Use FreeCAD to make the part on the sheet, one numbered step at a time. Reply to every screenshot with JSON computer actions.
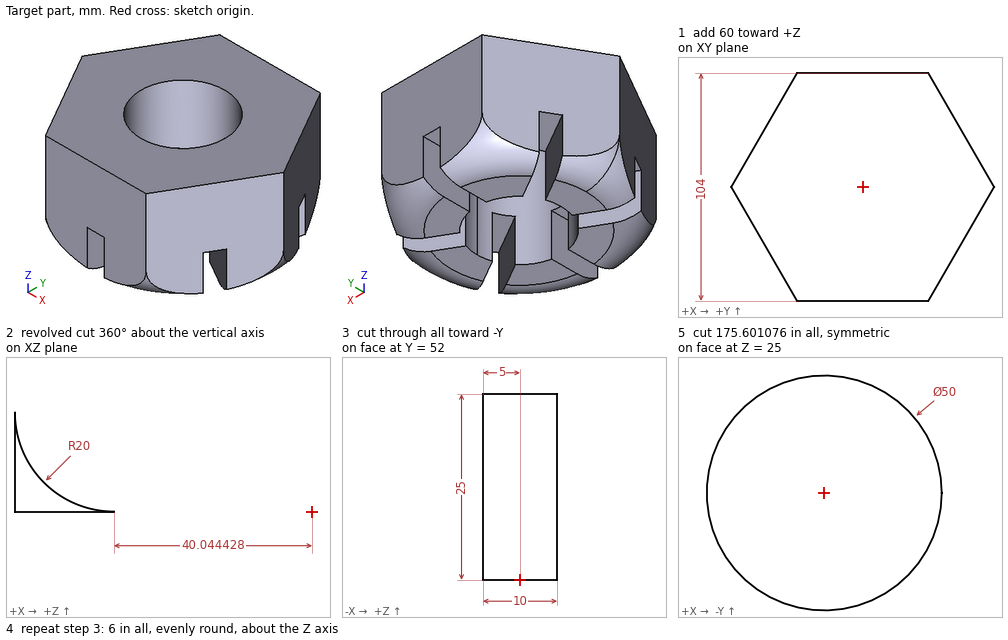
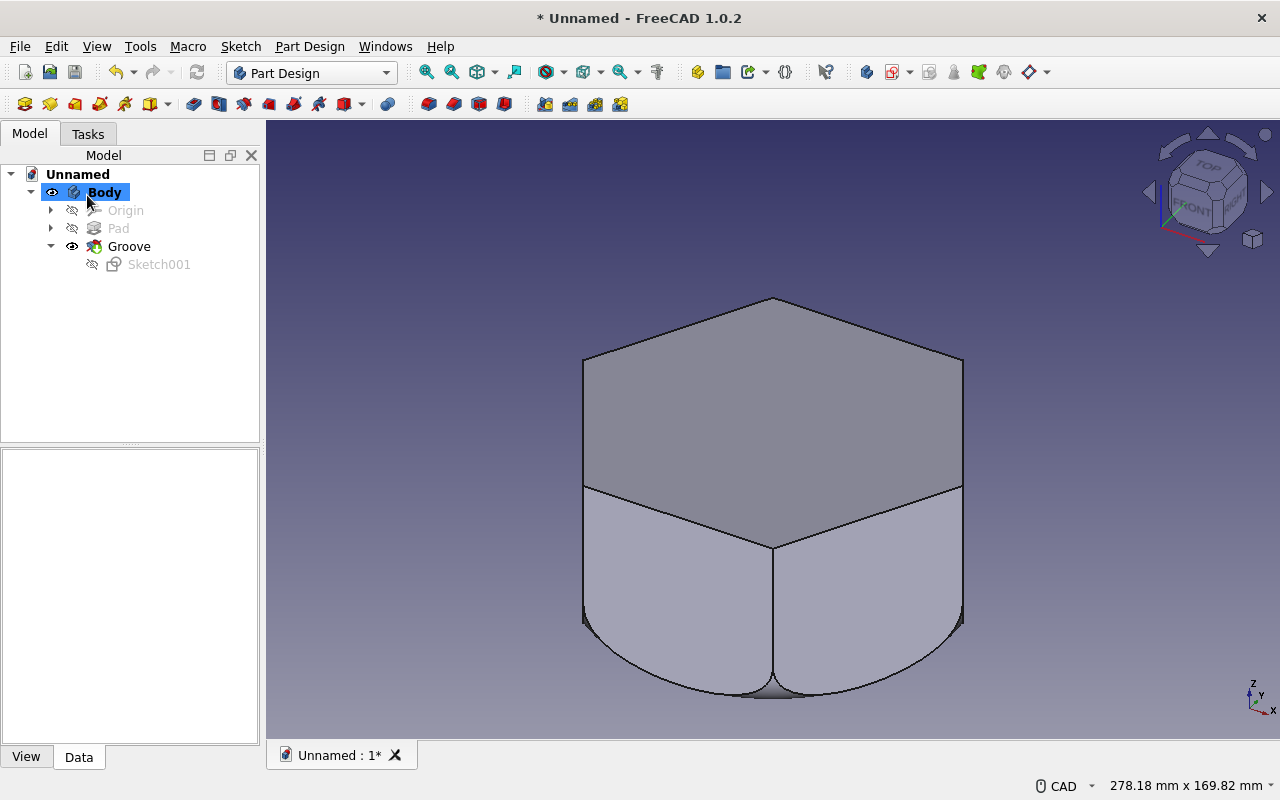
{"action": "left_click", "coordinate": [427, 72]}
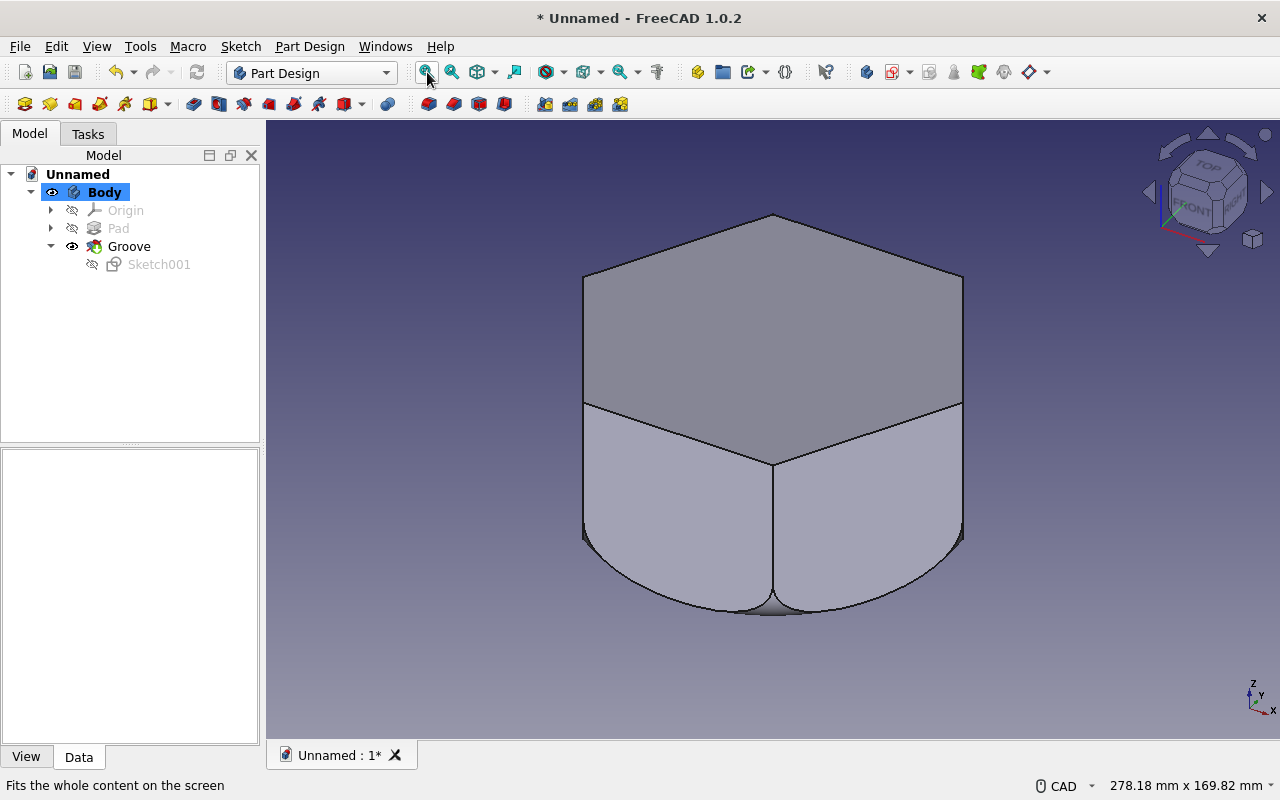
{"action": "key", "text": "4"}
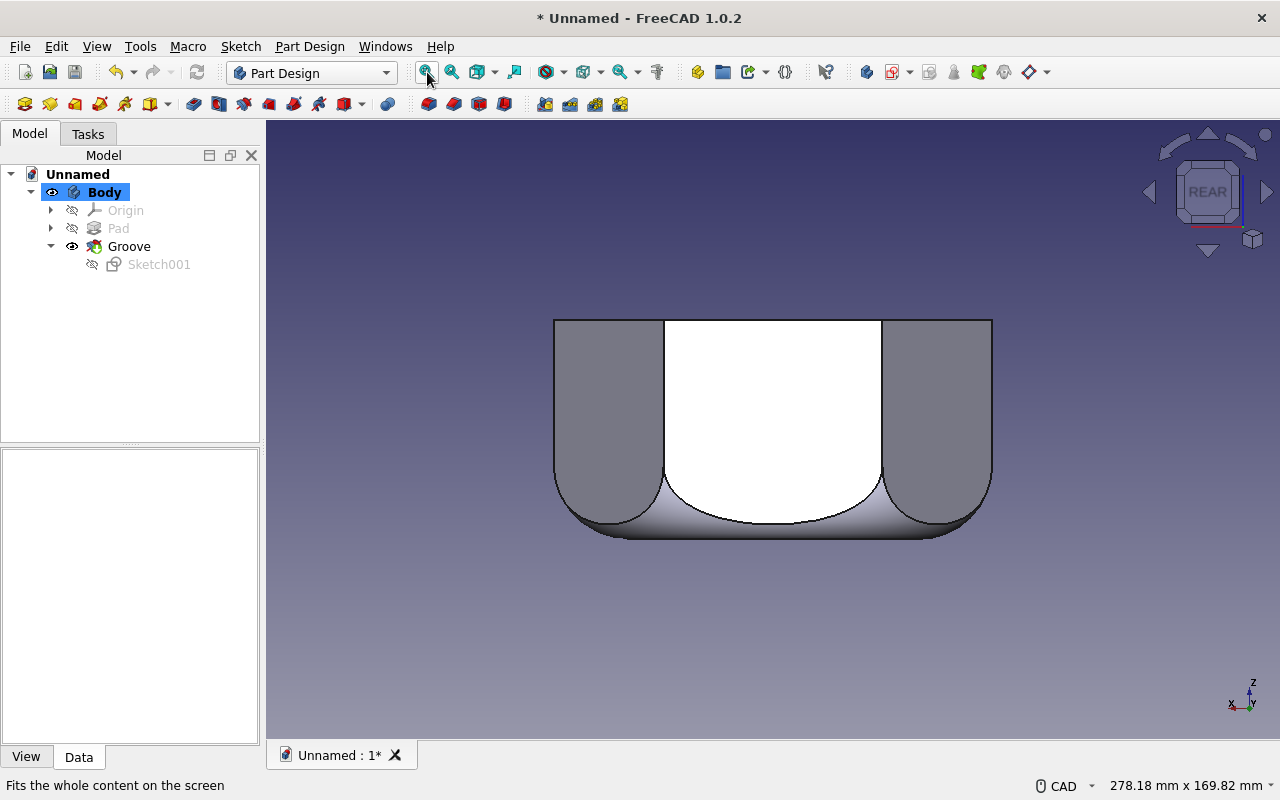
{"action": "left_click", "coordinate": [427, 72]}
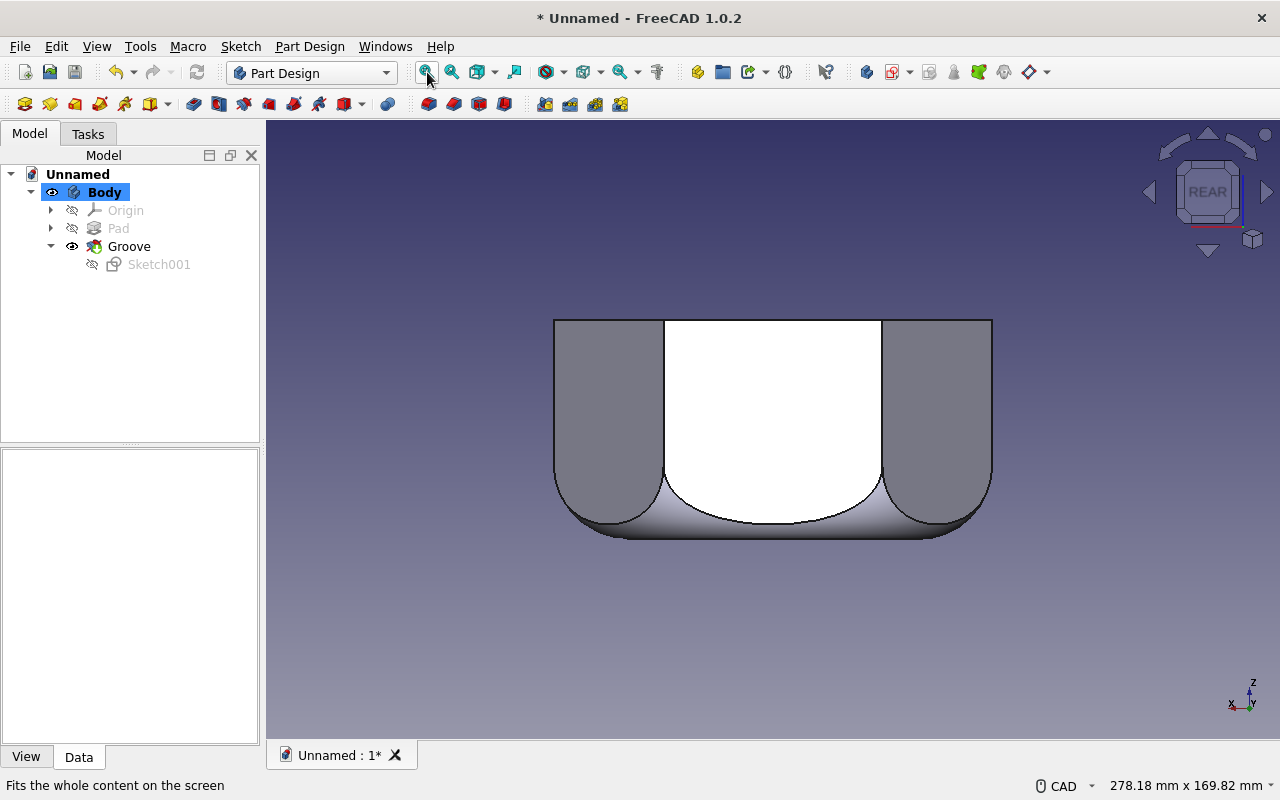
{"action": "left_click", "coordinate": [773, 421]}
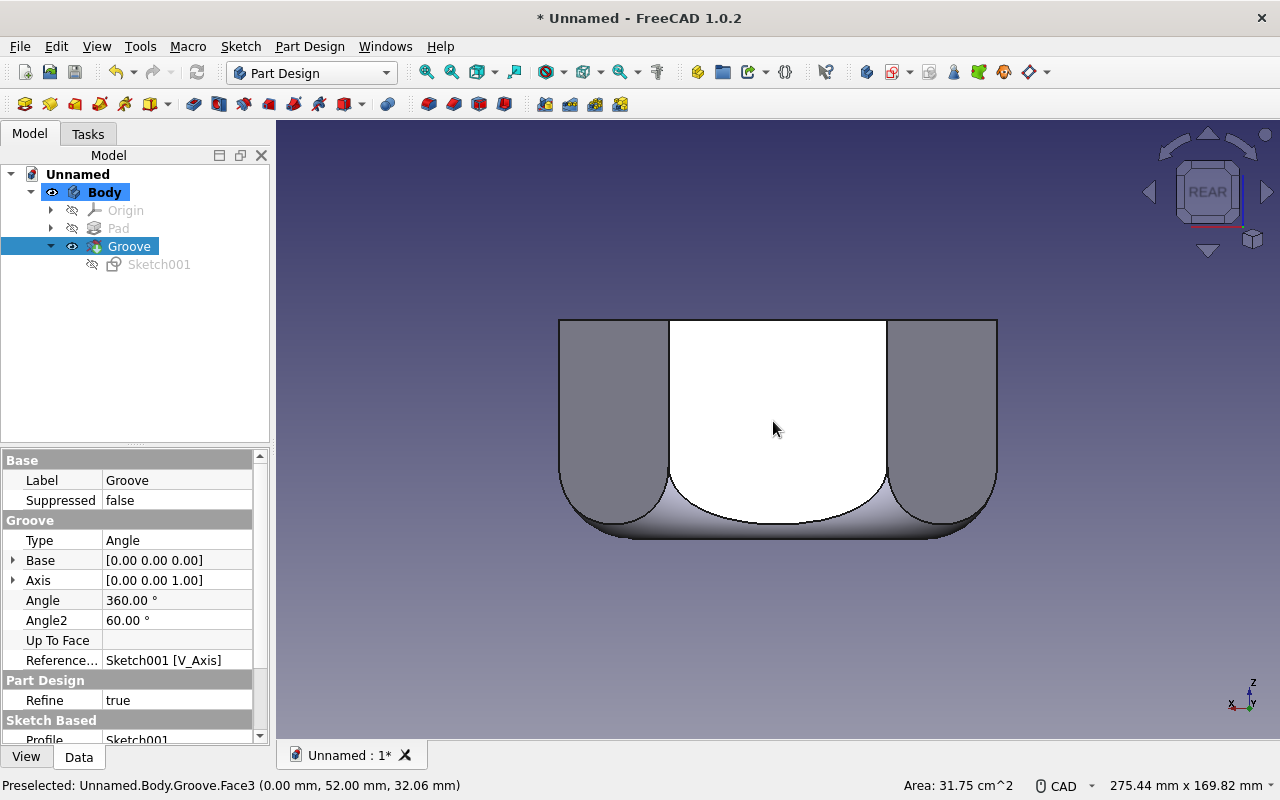
{"action": "left_click", "coordinate": [892, 72]}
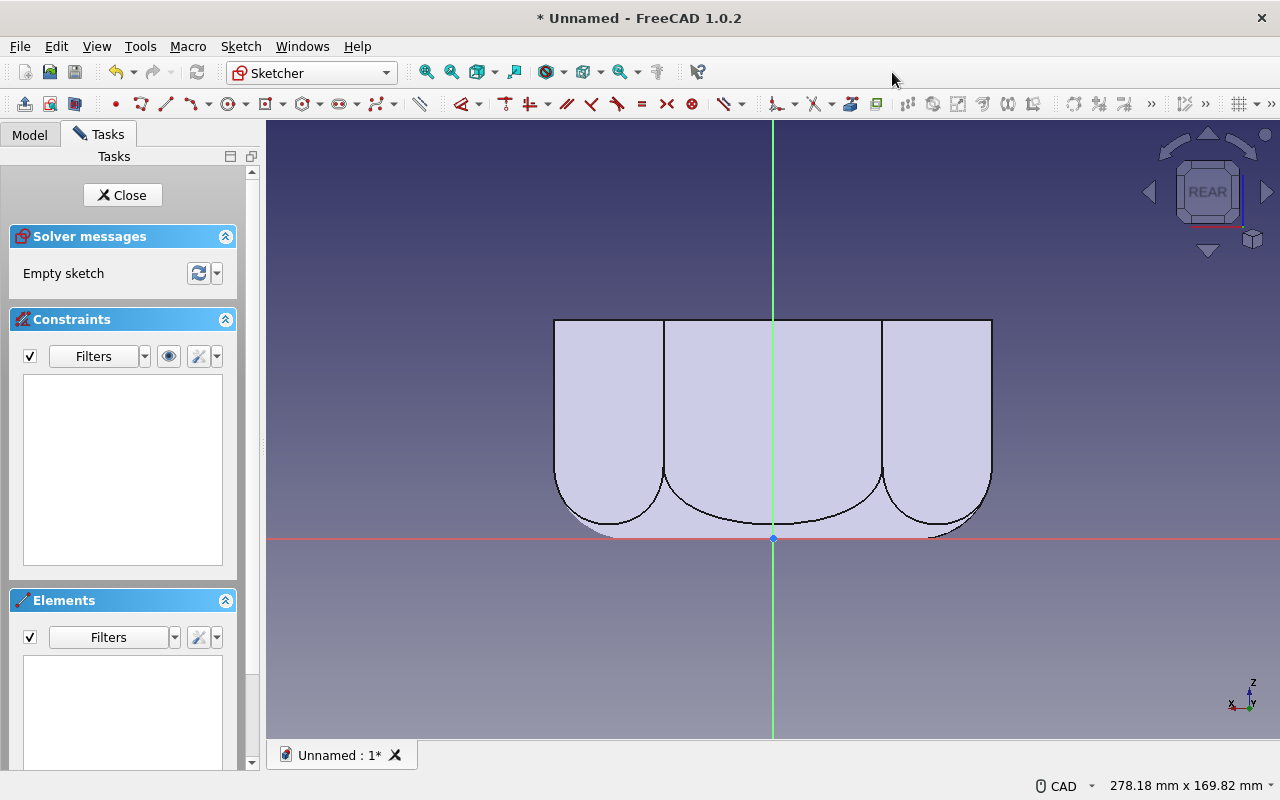
{"action": "scroll", "coordinate": [795, 514], "scroll_direction": "up", "scroll_amount": 7}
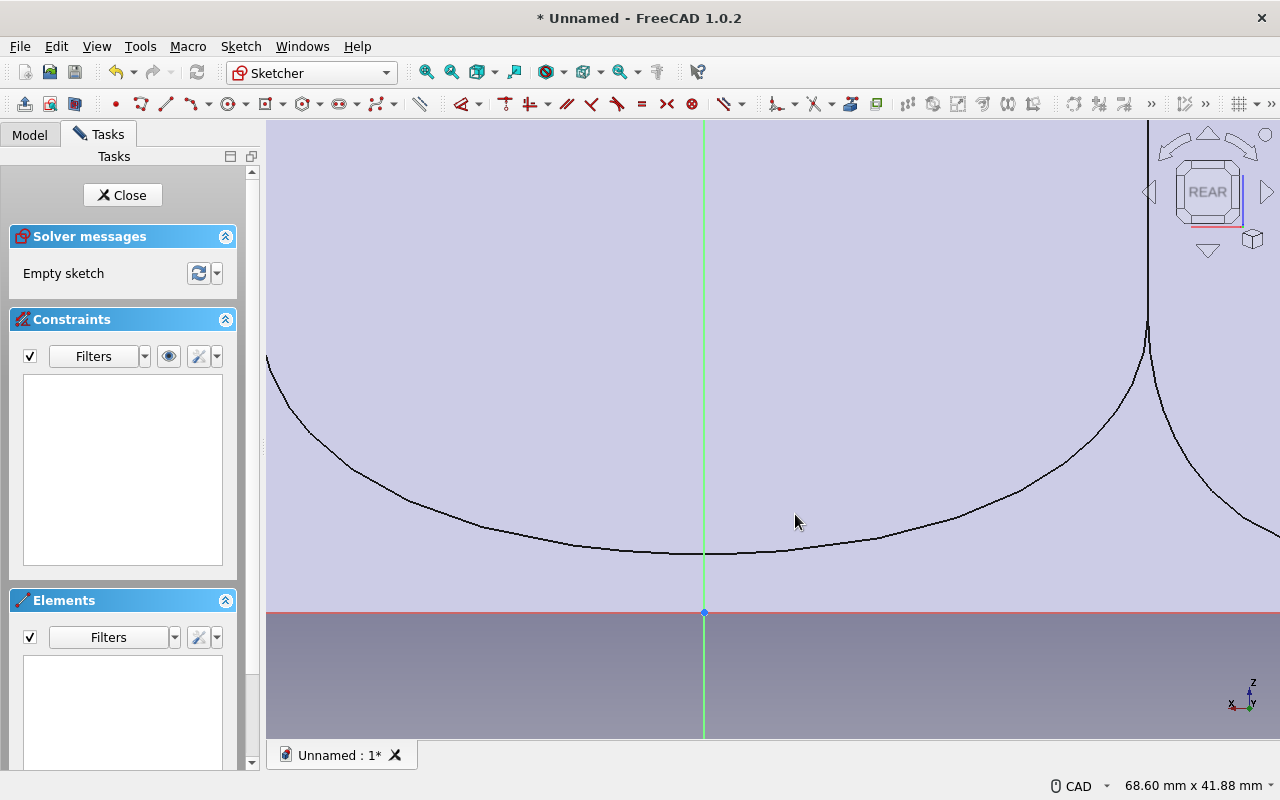
{"action": "key", "text": "g r"}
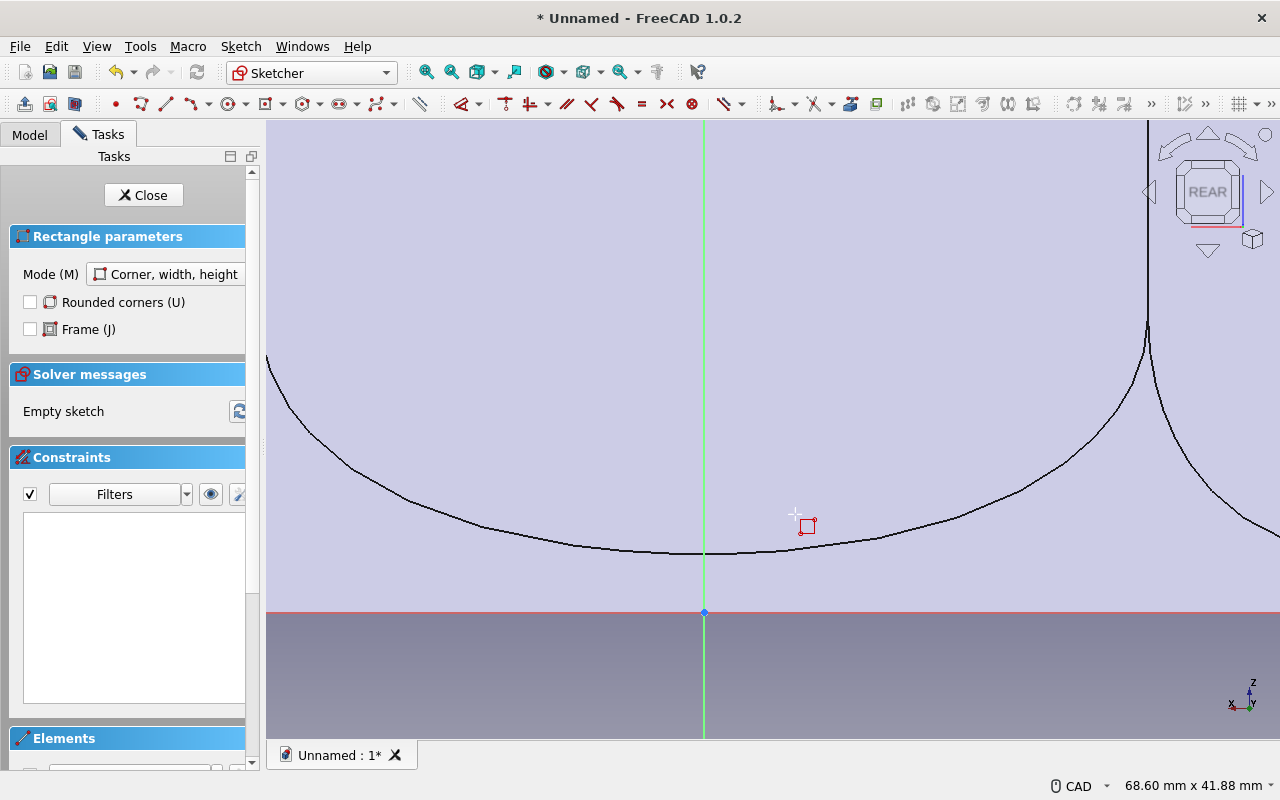
{"action": "left_click", "coordinate": [630, 243]}
{"action": "left_click", "coordinate": [778, 613]}
{"action": "key", "text": "Escape"}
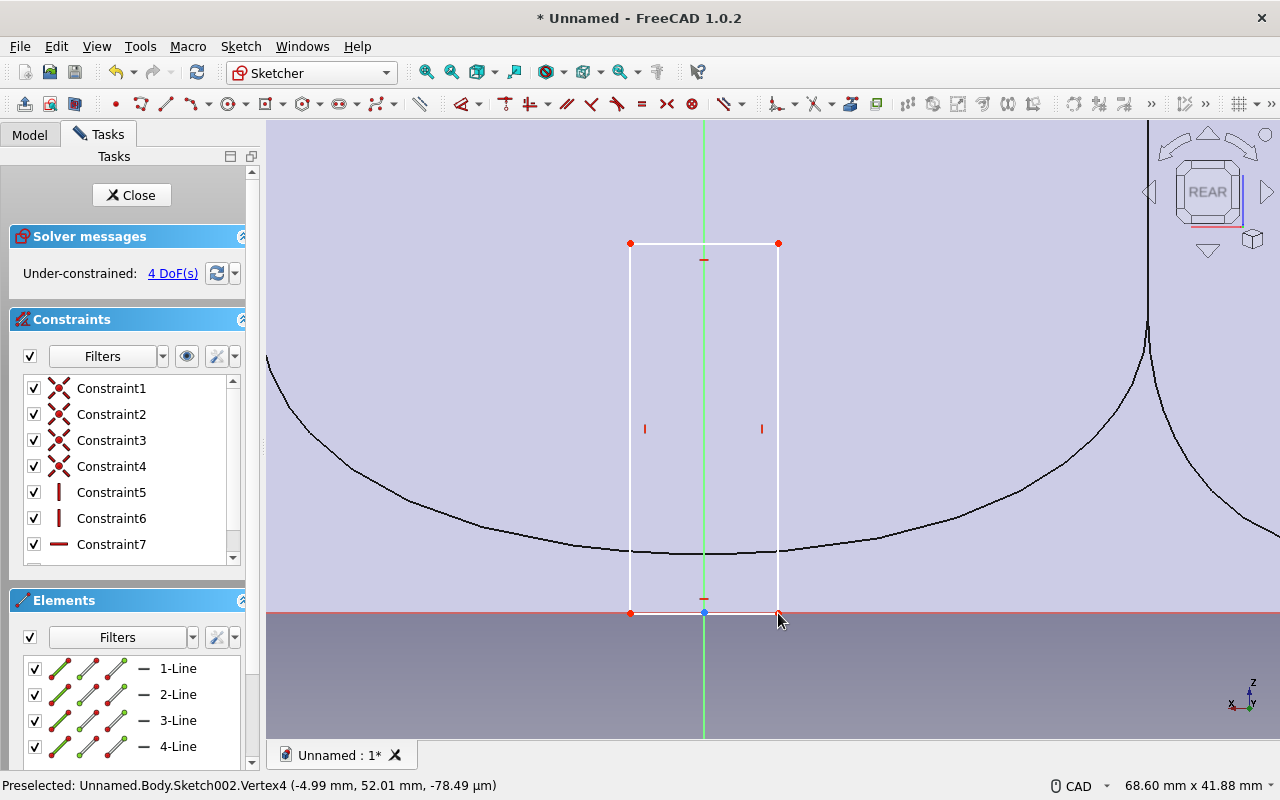
{"action": "left_click", "coordinate": [630, 614]}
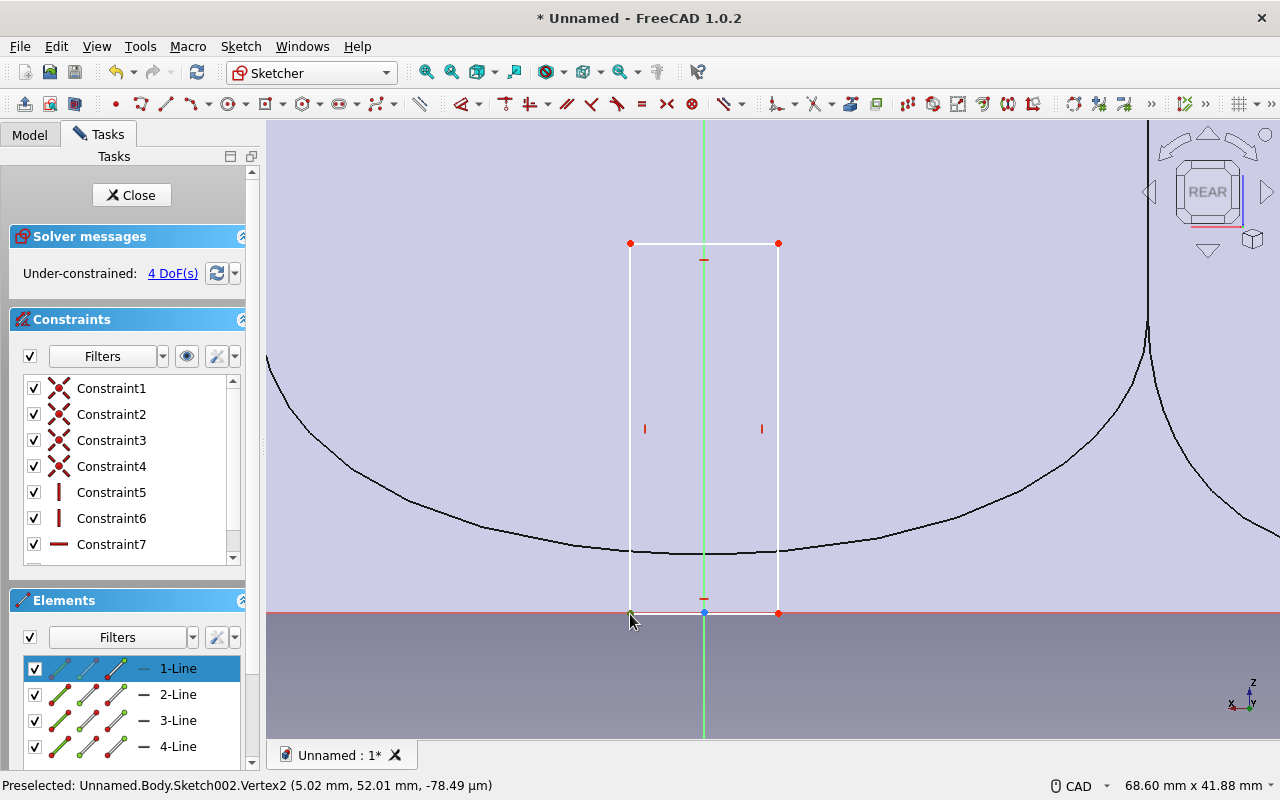
{"action": "left_click", "coordinate": [353, 613]}